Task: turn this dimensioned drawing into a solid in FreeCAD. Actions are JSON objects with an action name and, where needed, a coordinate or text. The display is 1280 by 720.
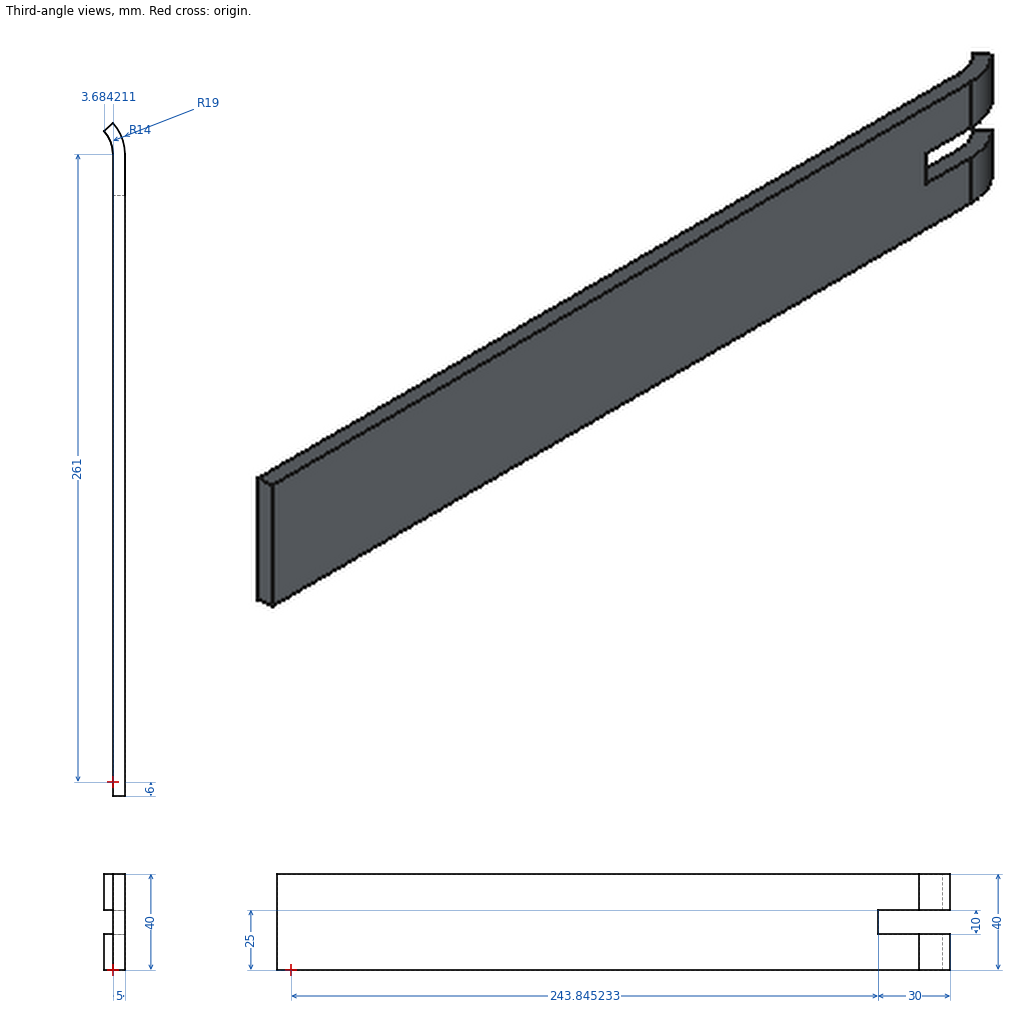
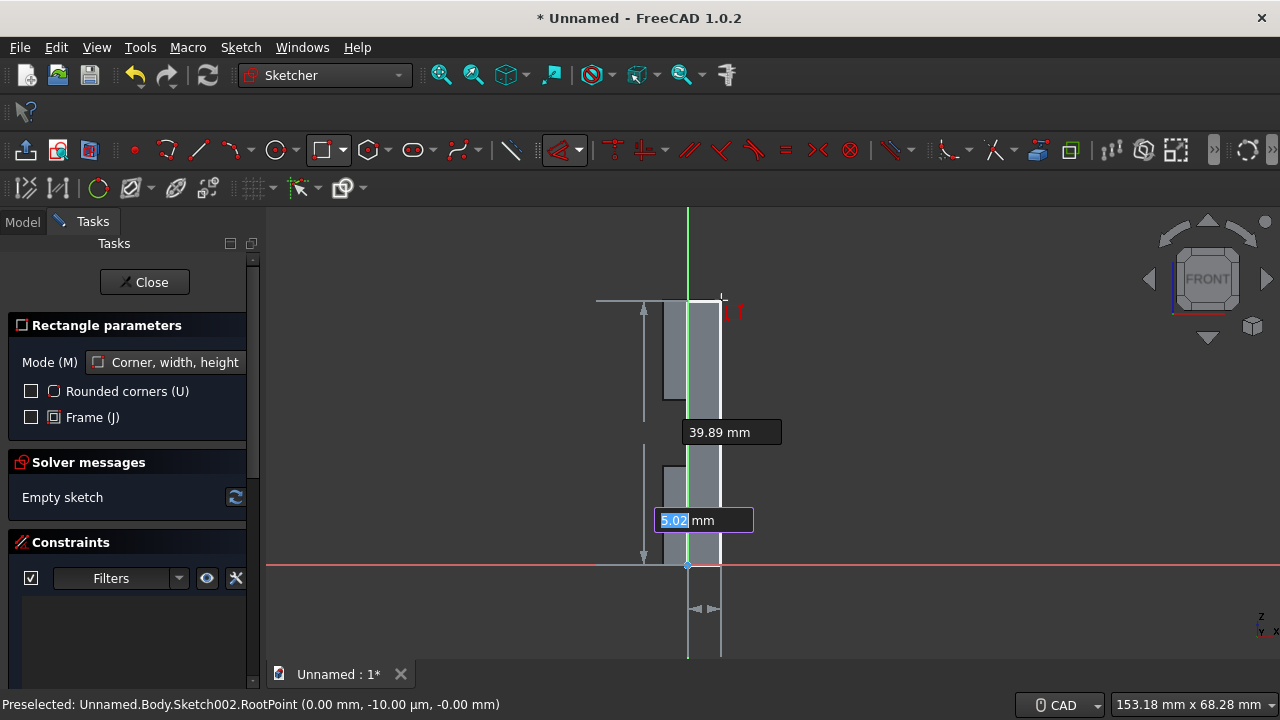
{"action": "type", "text": "5"}
{"action": "key", "text": "Tab"}
{"action": "type", "text": "40"}
{"action": "key", "text": "Return"}
{"action": "key", "text": "Escape"}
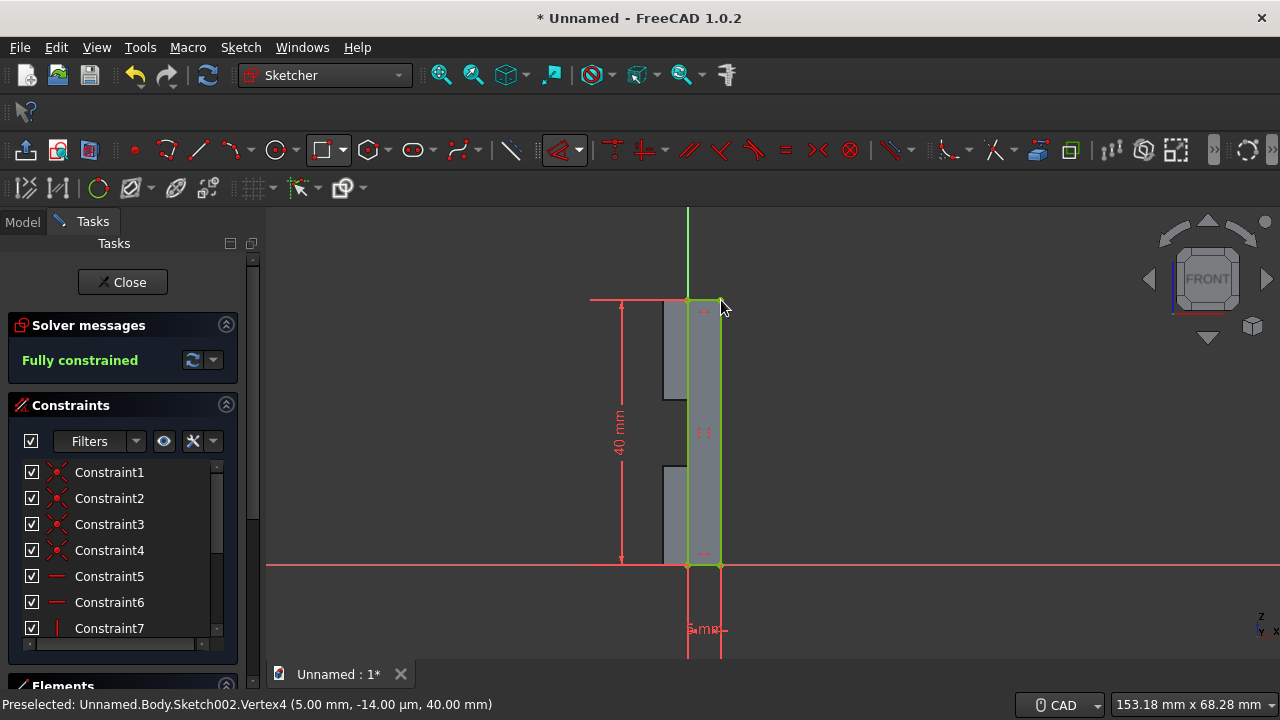
{"action": "left_click", "coordinate": [123, 282]}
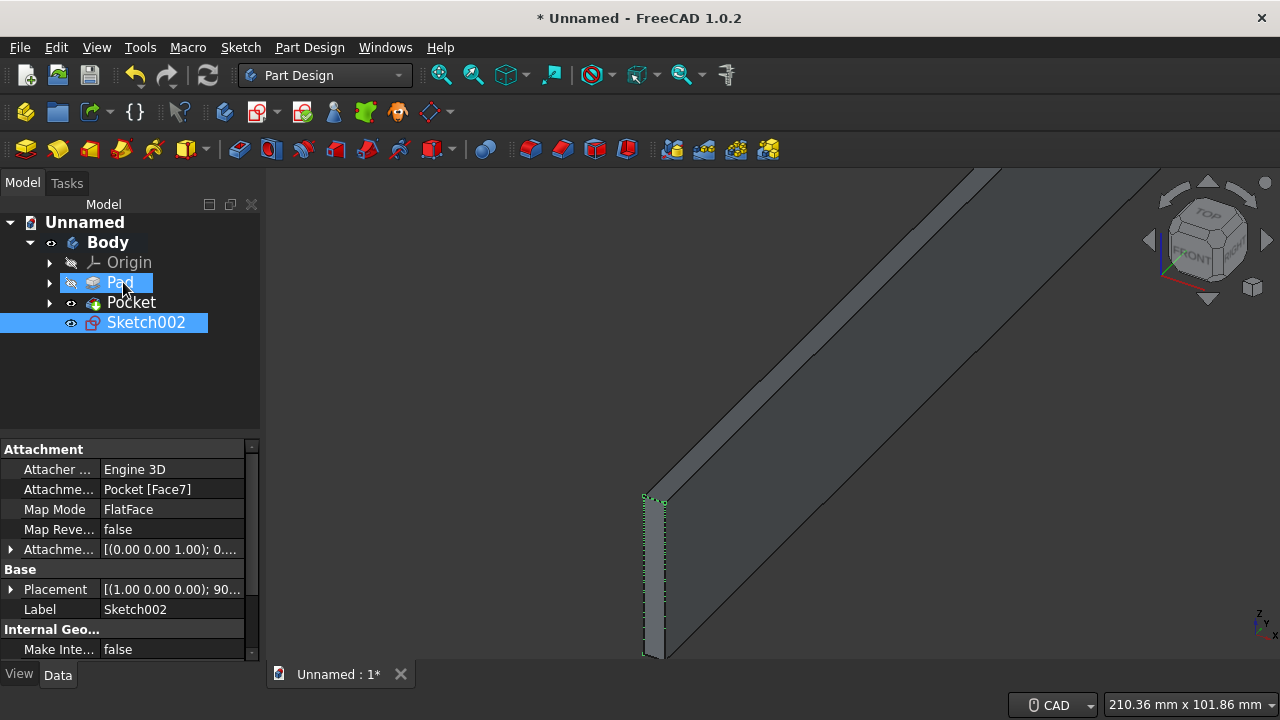
{"action": "left_click", "coordinate": [26, 150]}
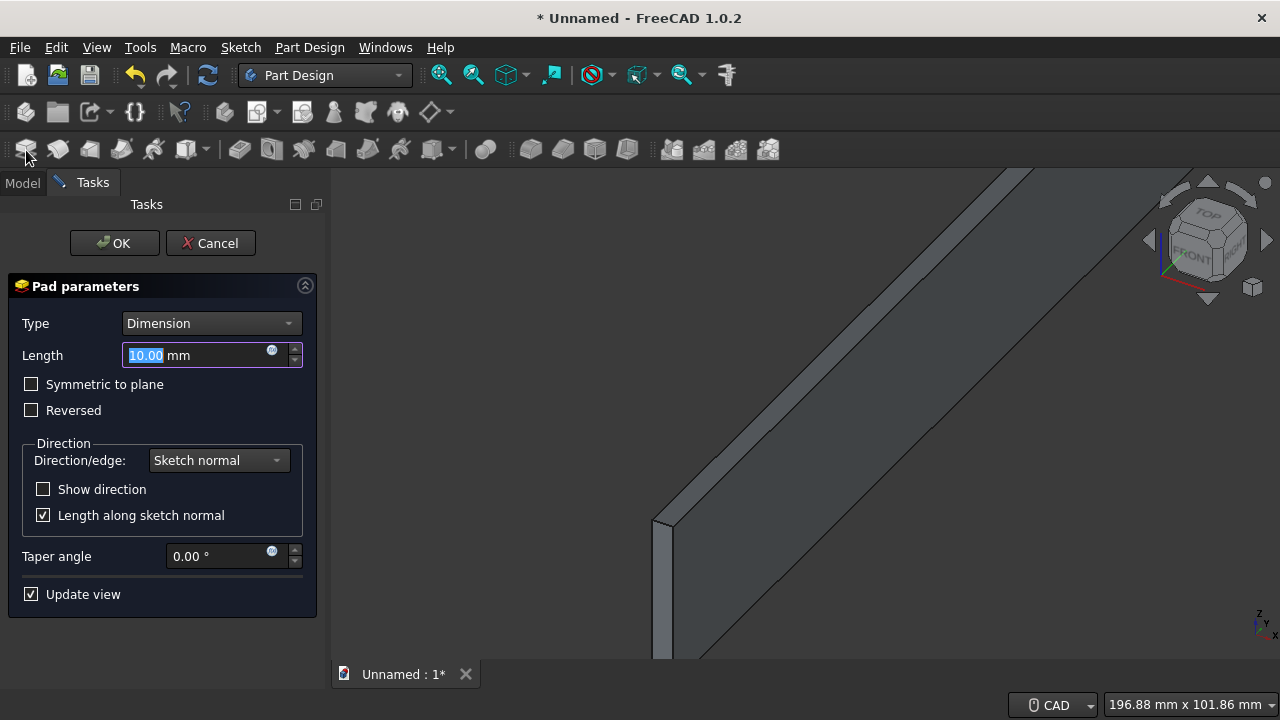
{"action": "type", "text": "6"}
{"action": "key", "text": "Tab"}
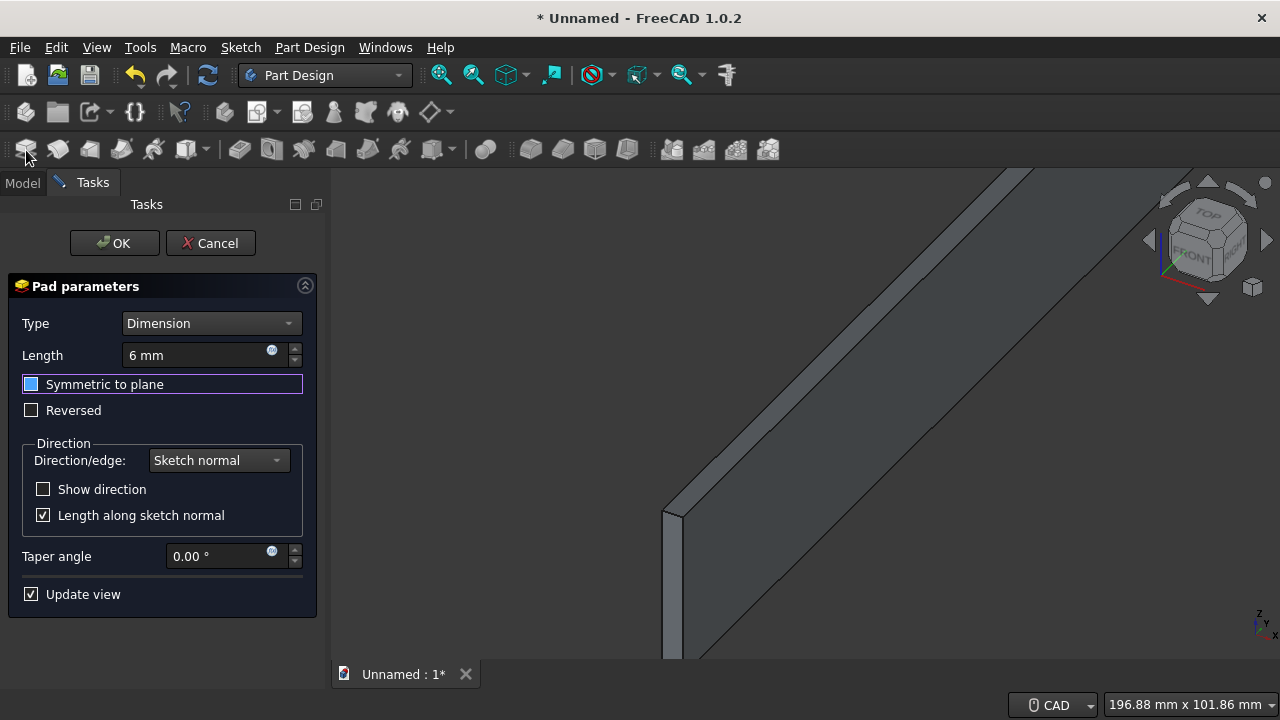
{"action": "left_click", "coordinate": [115, 243]}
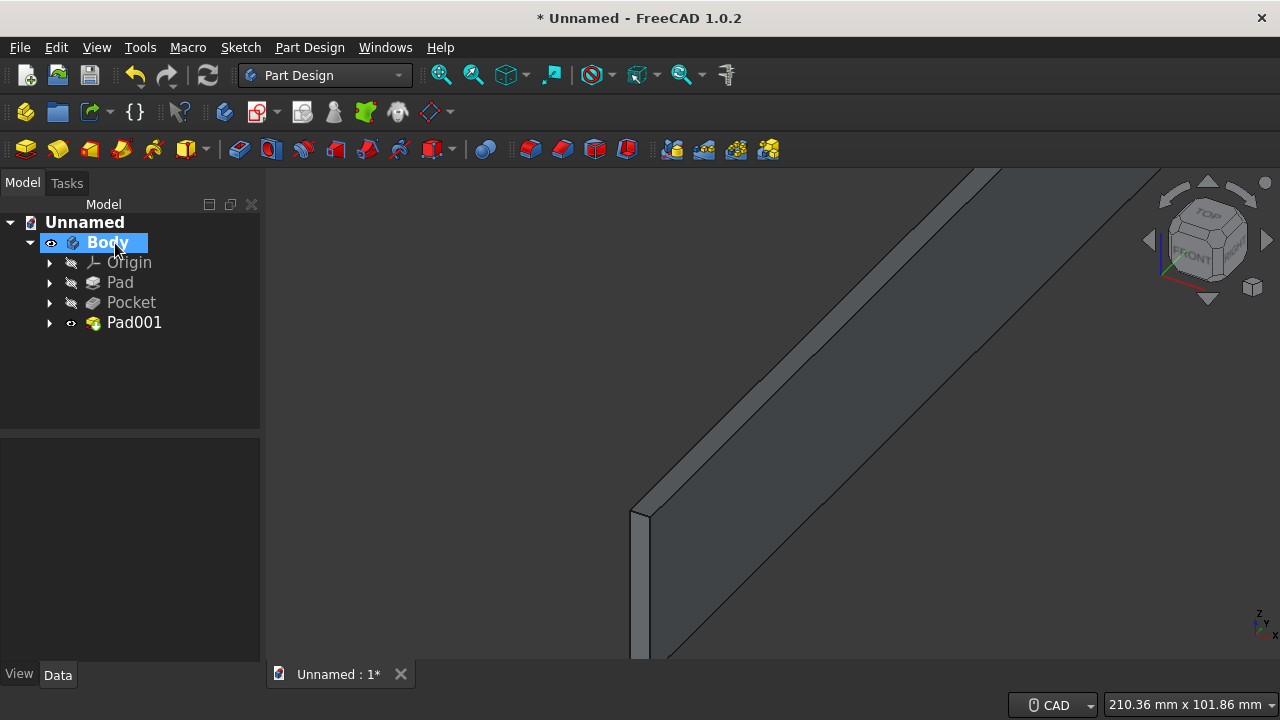
{"action": "key", "text": "0"}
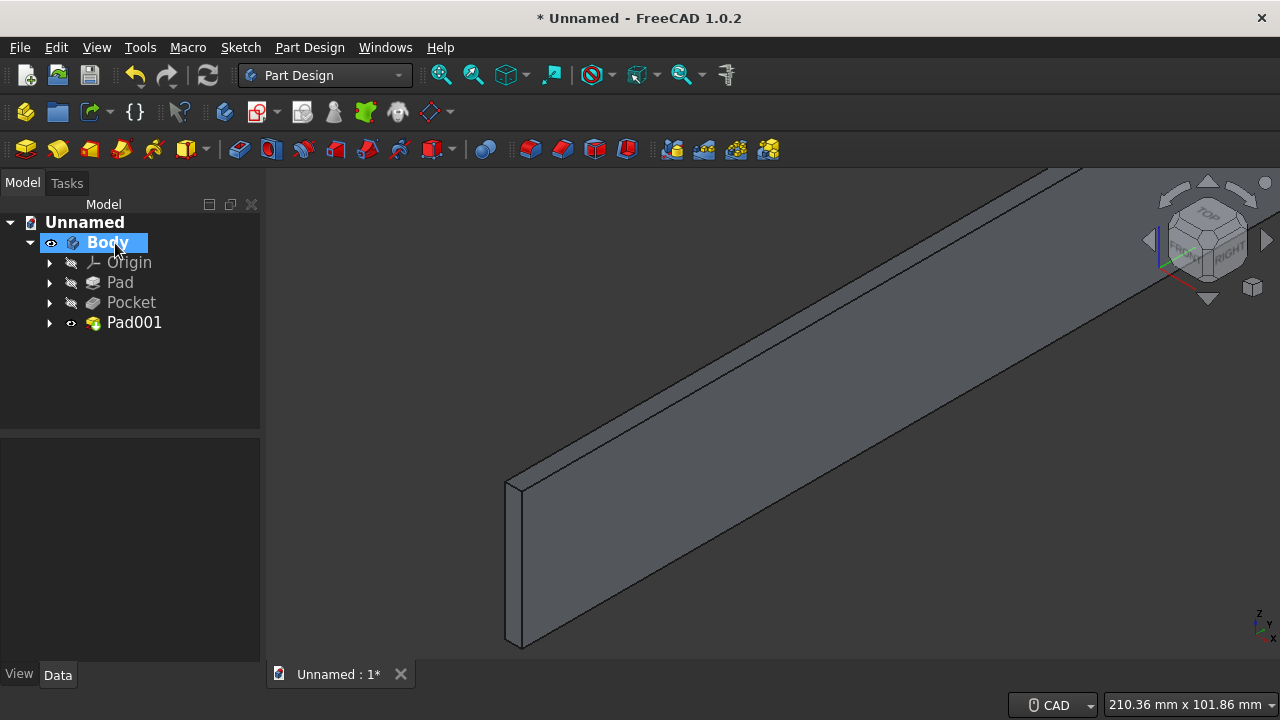
{"action": "left_click", "coordinate": [442, 76]}